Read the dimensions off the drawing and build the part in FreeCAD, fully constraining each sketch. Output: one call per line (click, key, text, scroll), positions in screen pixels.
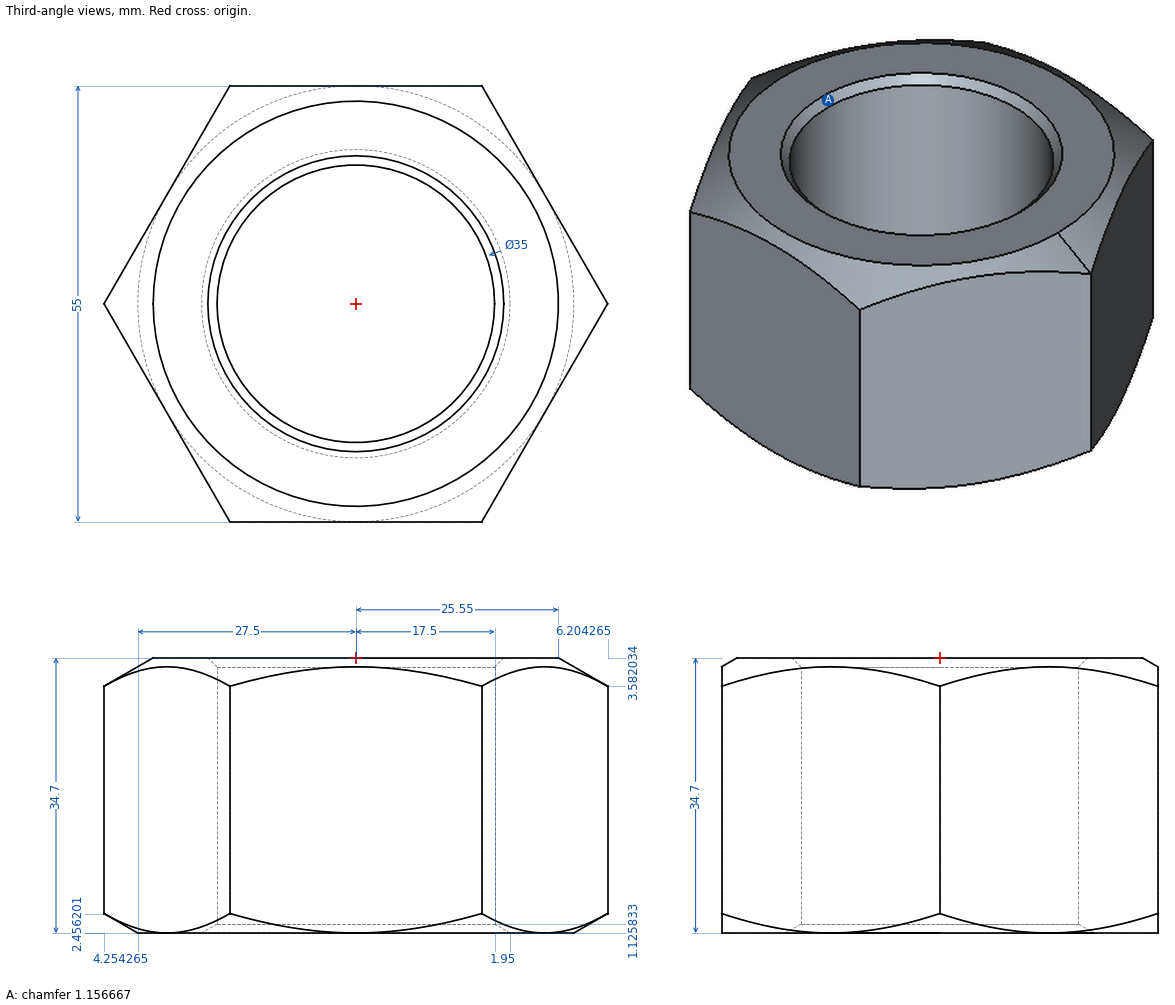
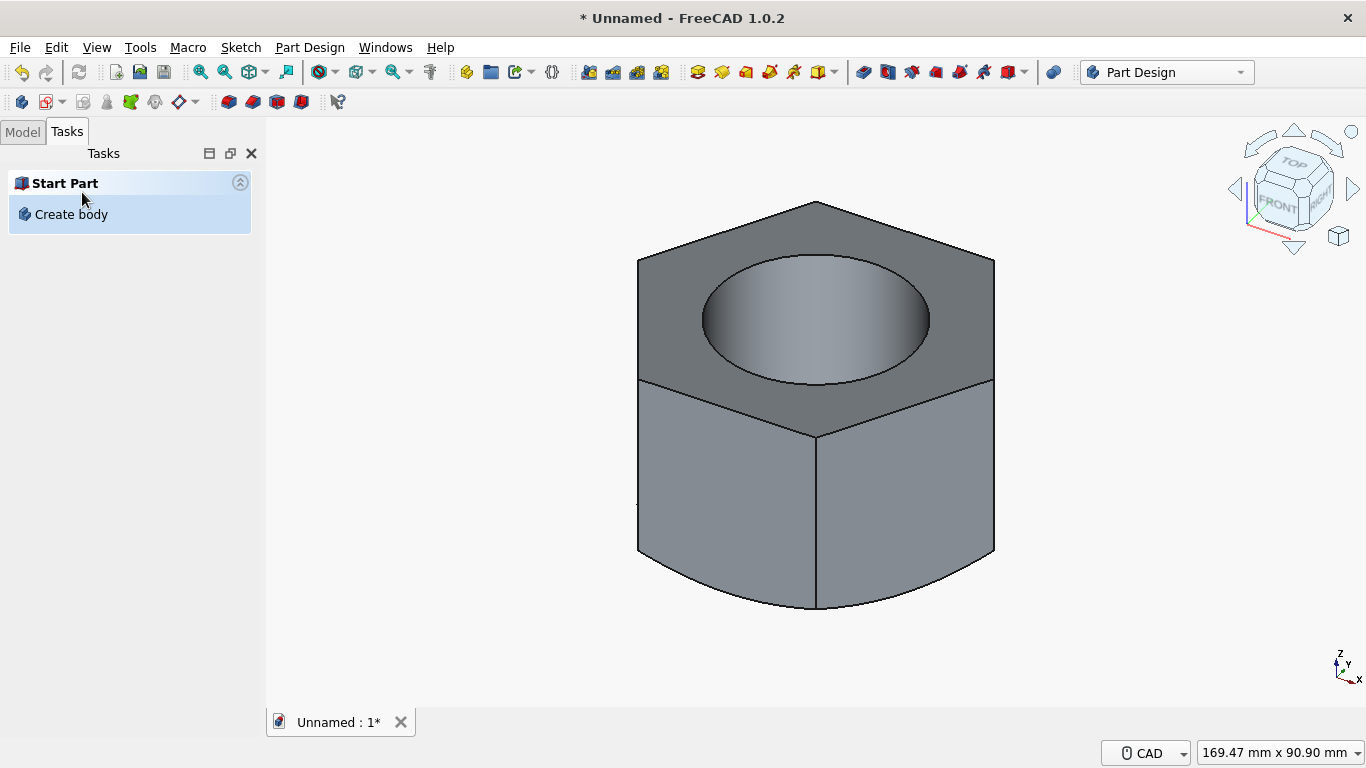
click(46, 102)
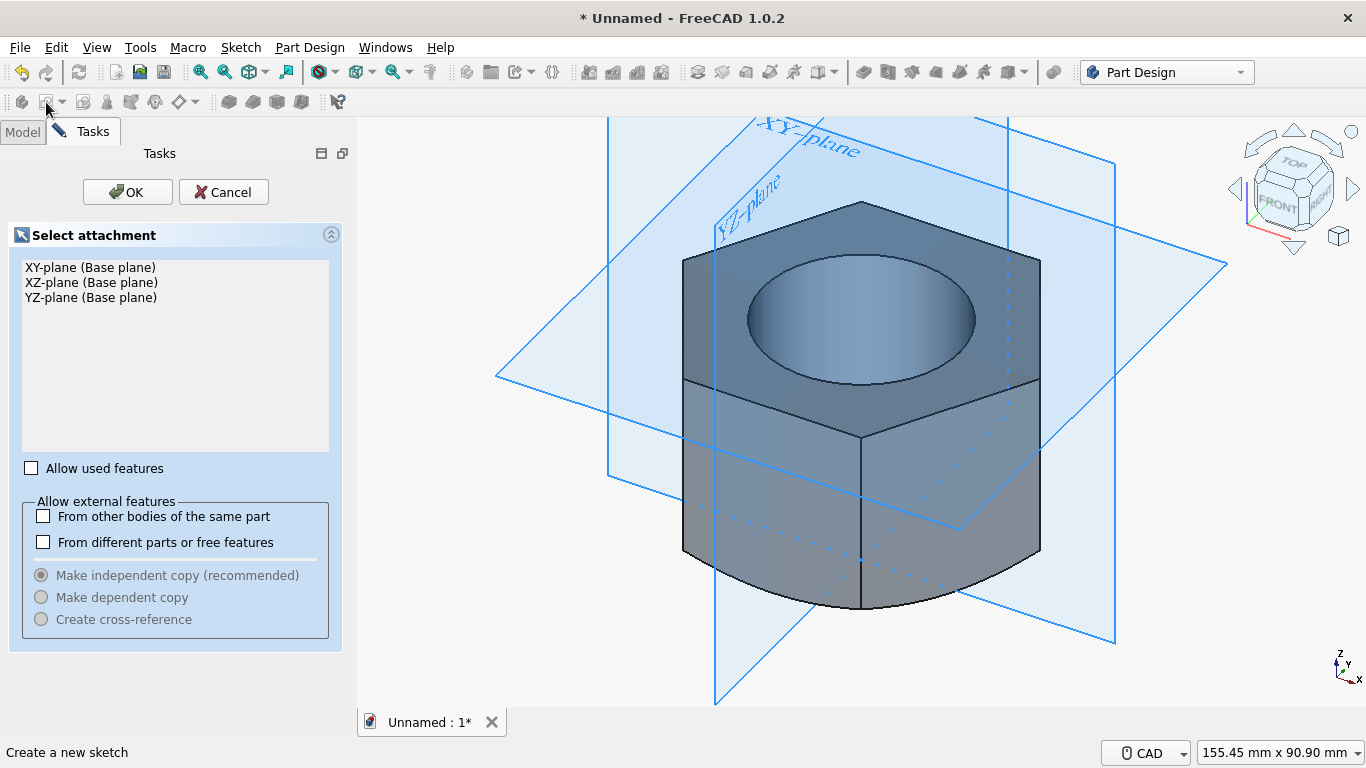
click(82, 282)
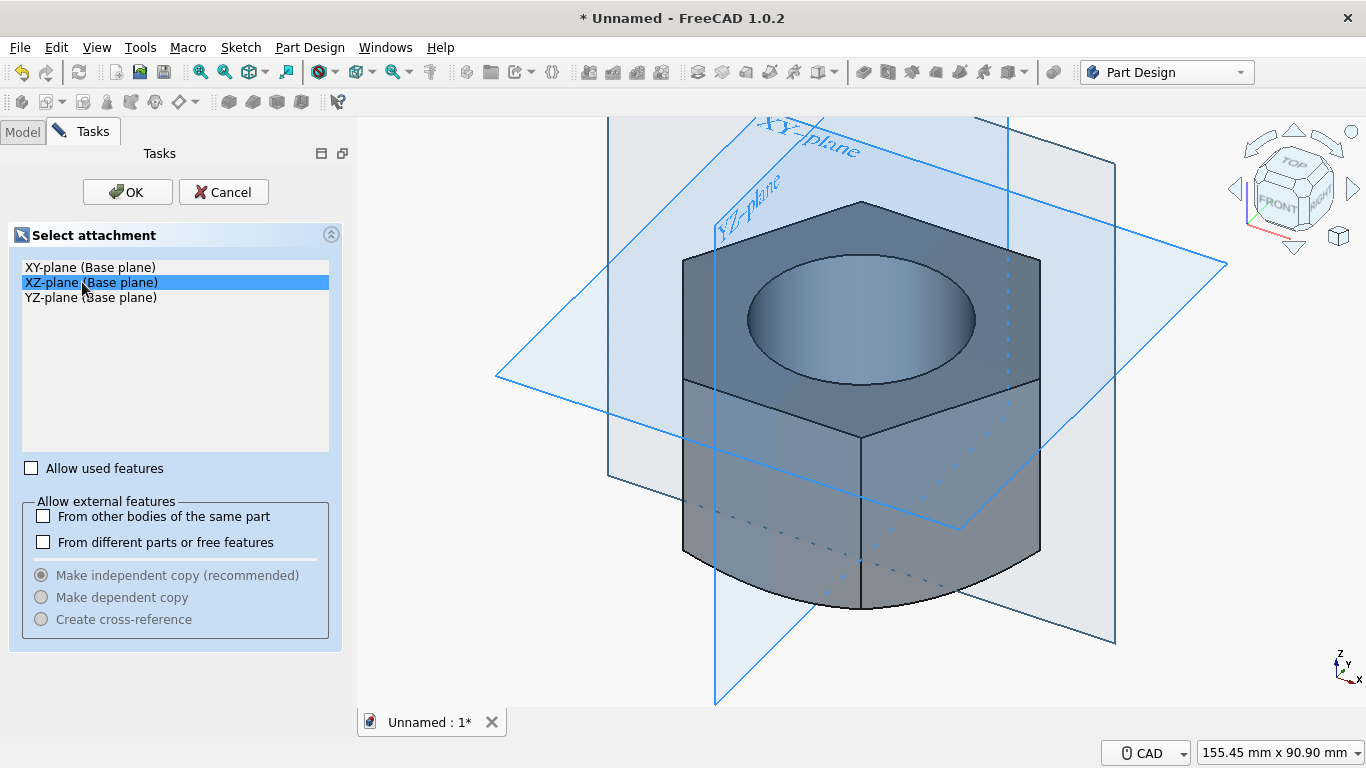
click(128, 192)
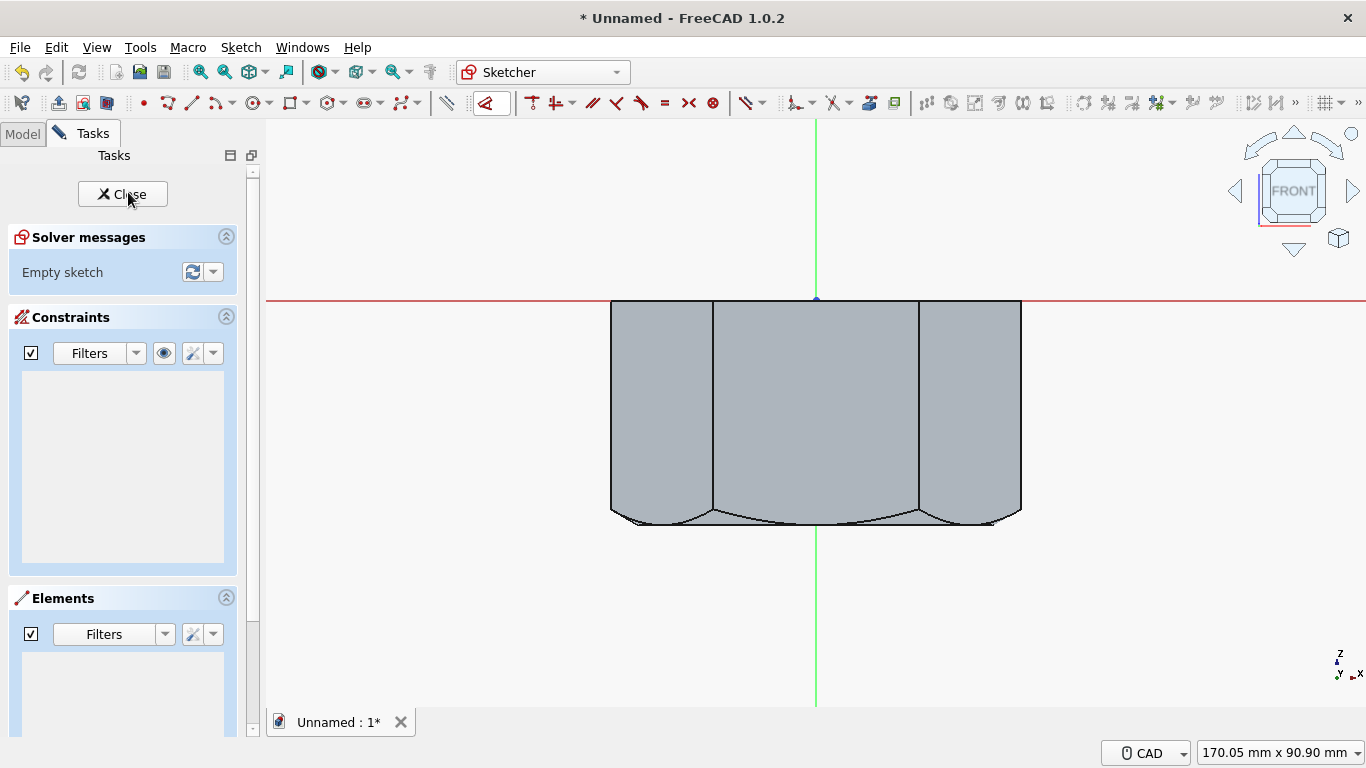
click(108, 104)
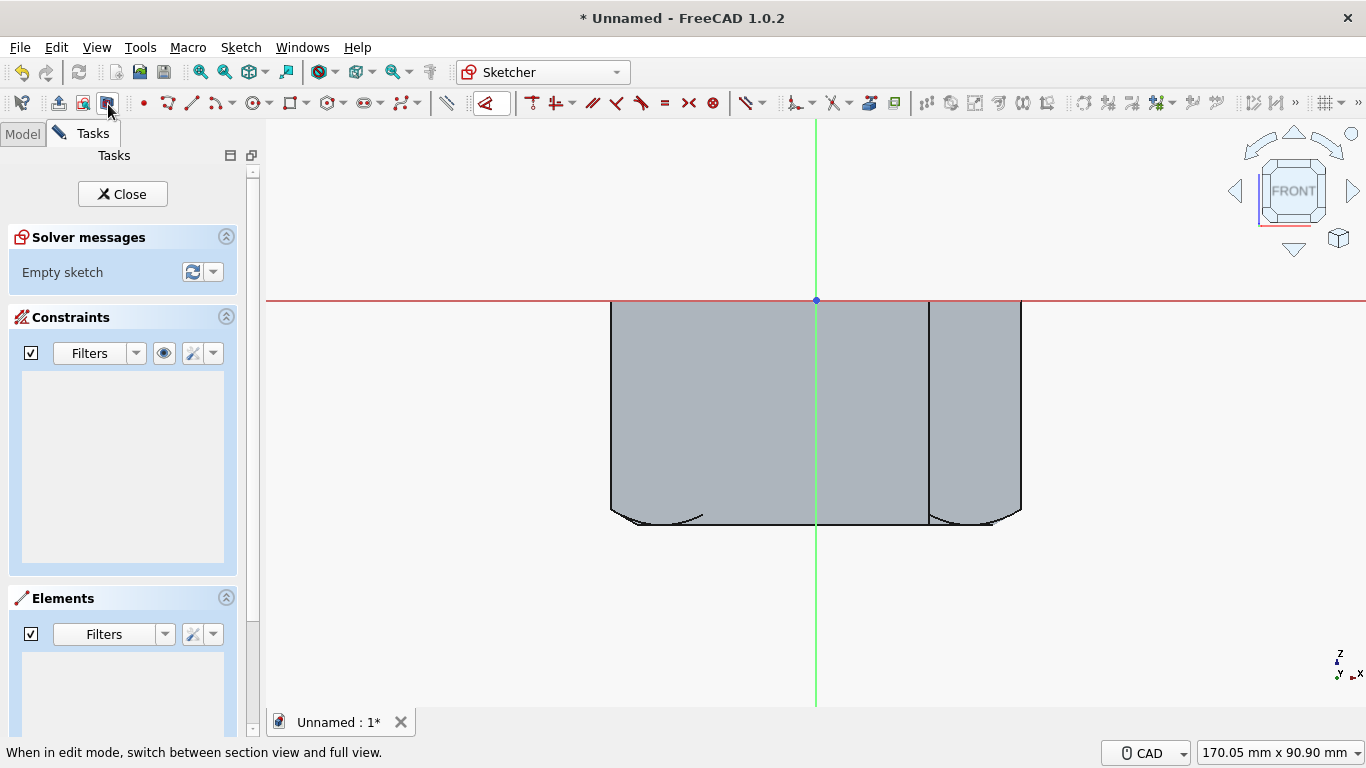
scroll(945, 527, up, 15)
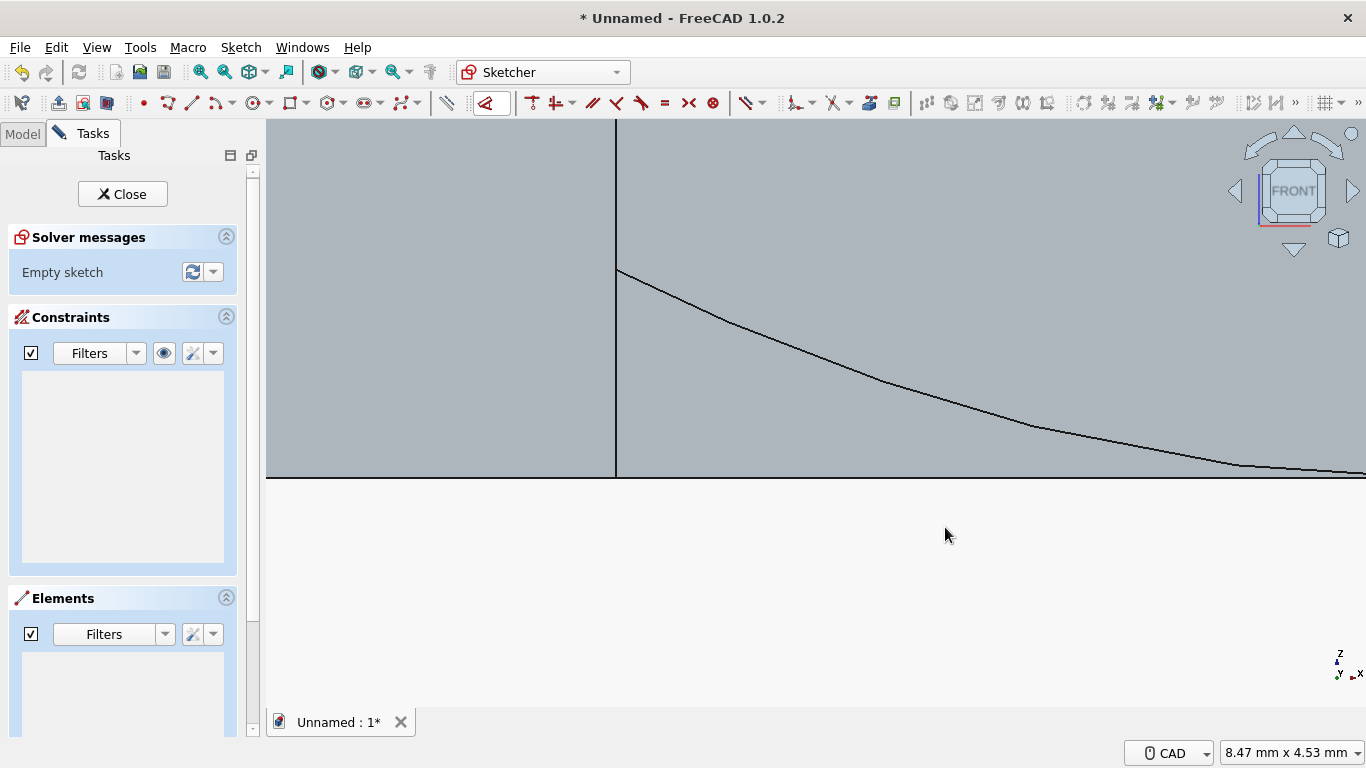
scroll(740, 401, up, 5)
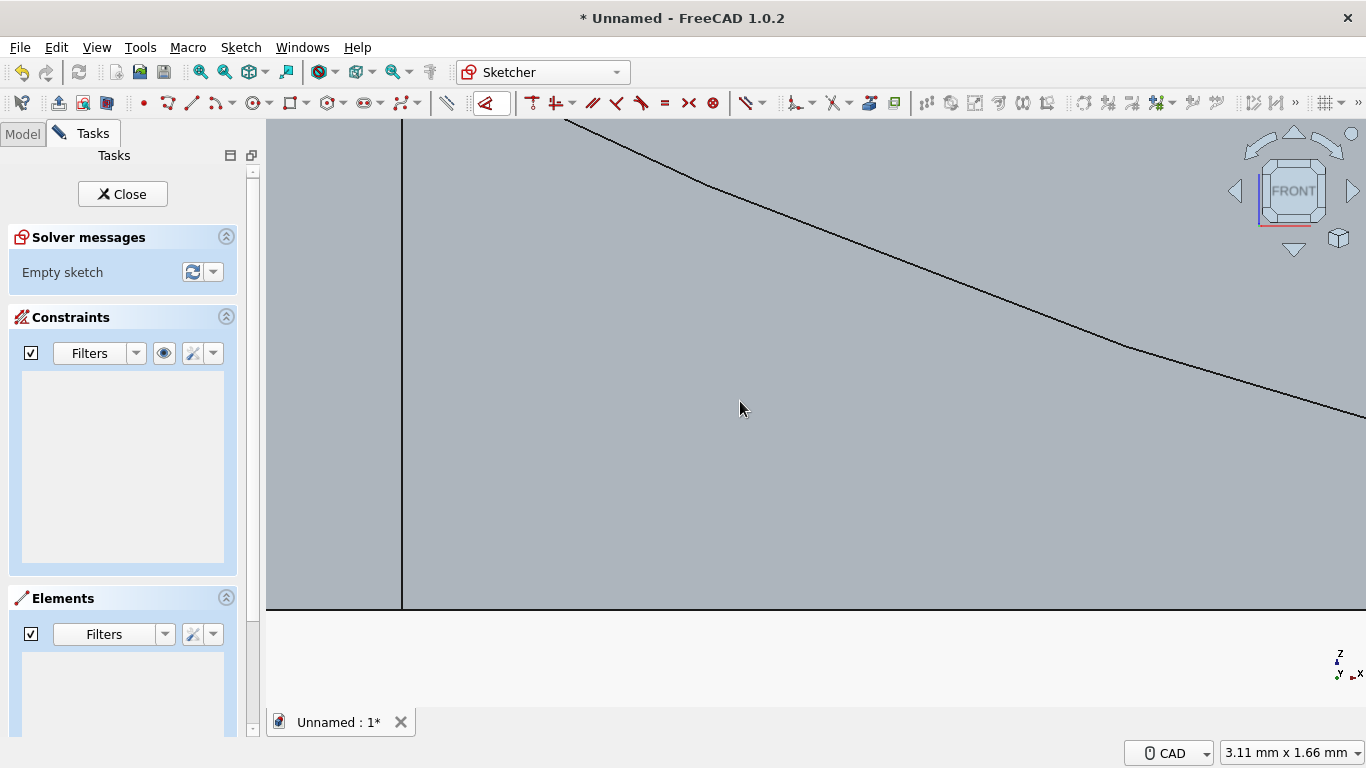
key(g)
key(m)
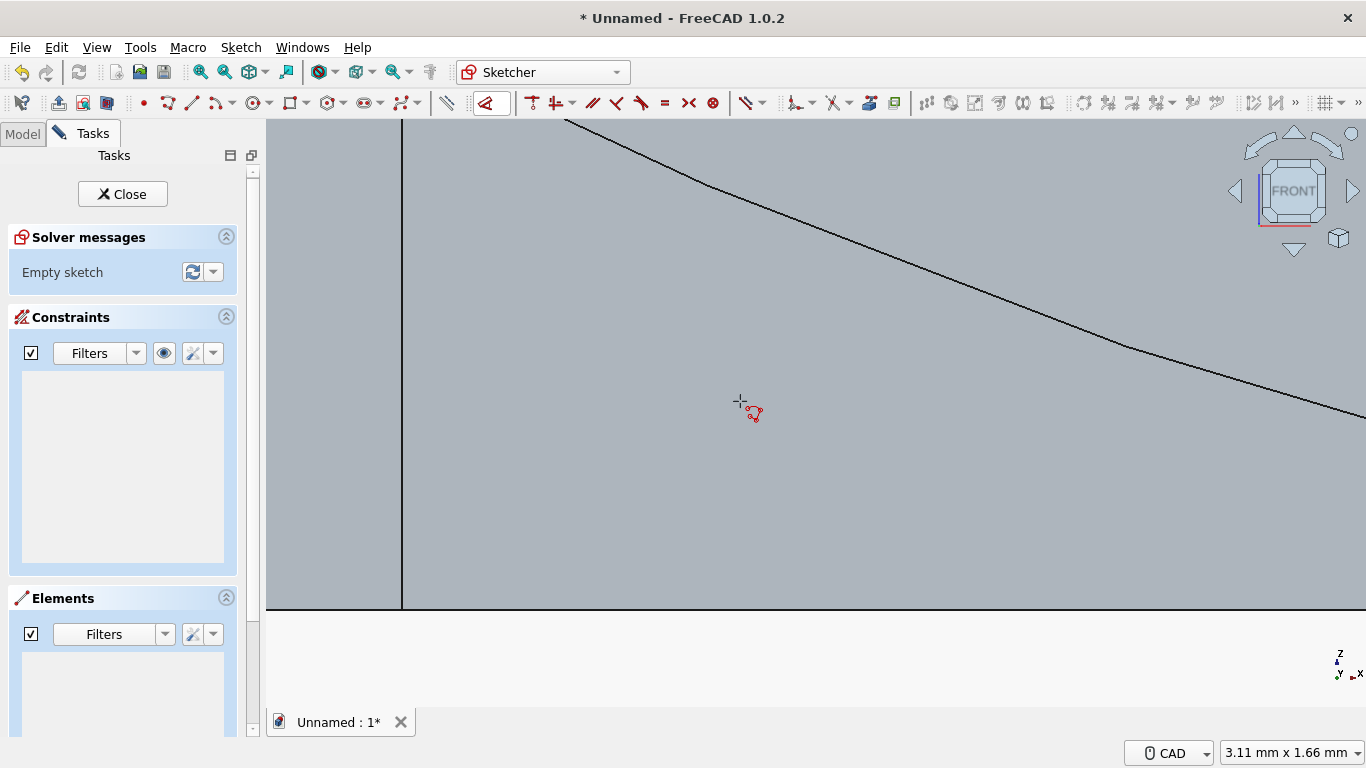
click(402, 213)
click(1091, 610)
click(402, 610)
click(402, 214)
key(Escape)
key(Escape)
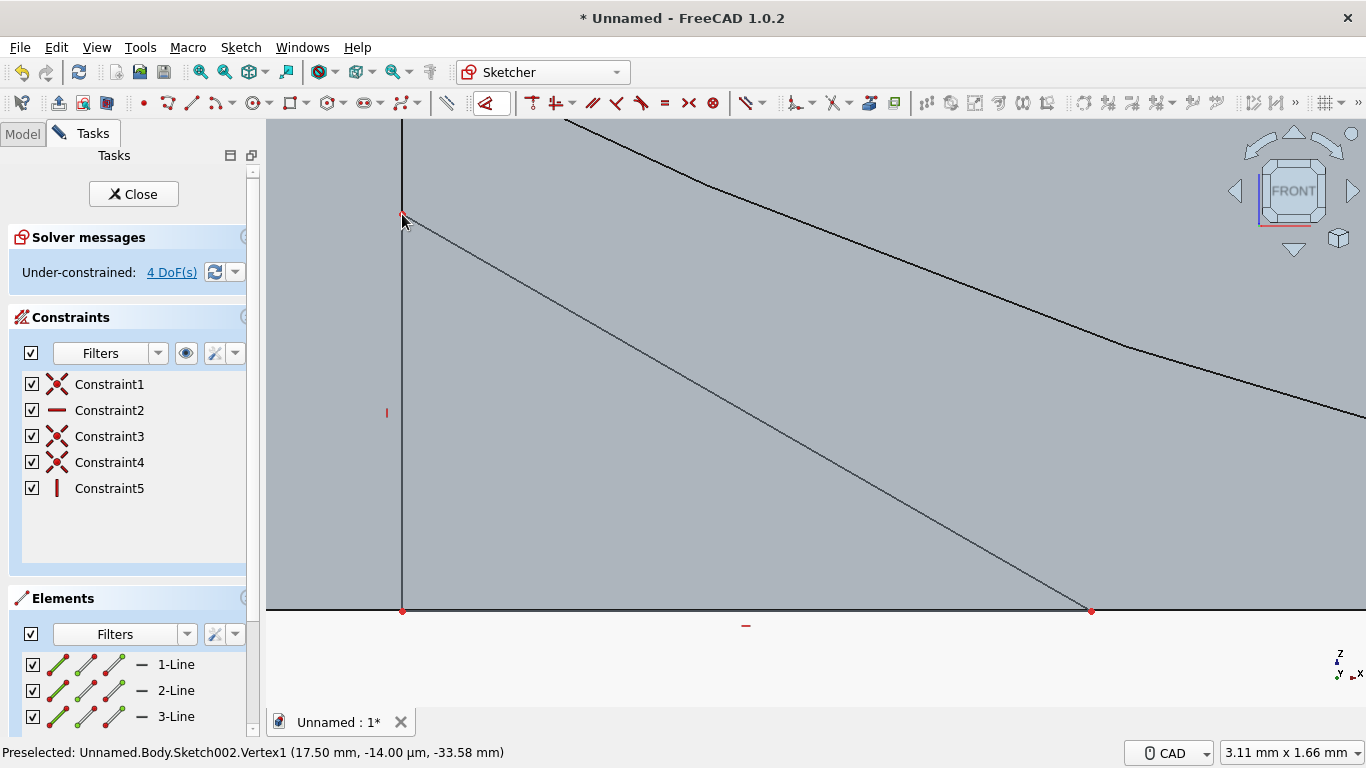
click(884, 611)